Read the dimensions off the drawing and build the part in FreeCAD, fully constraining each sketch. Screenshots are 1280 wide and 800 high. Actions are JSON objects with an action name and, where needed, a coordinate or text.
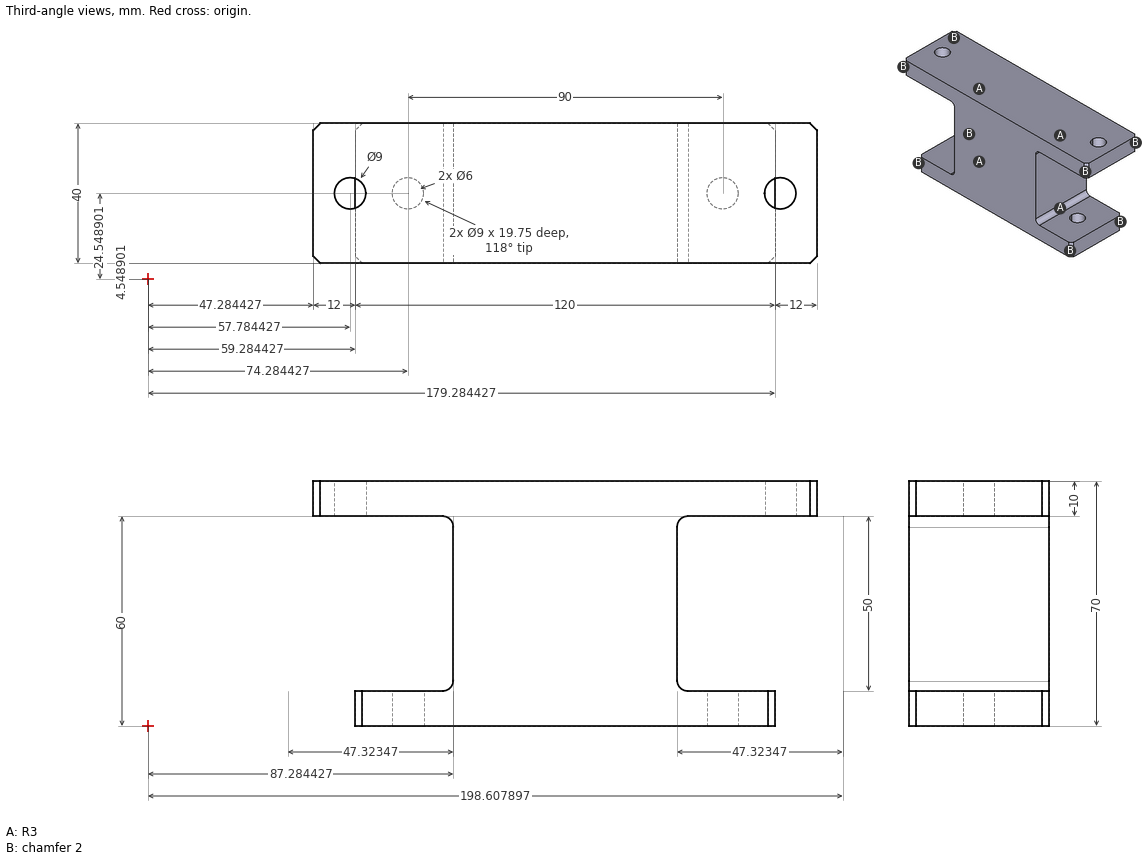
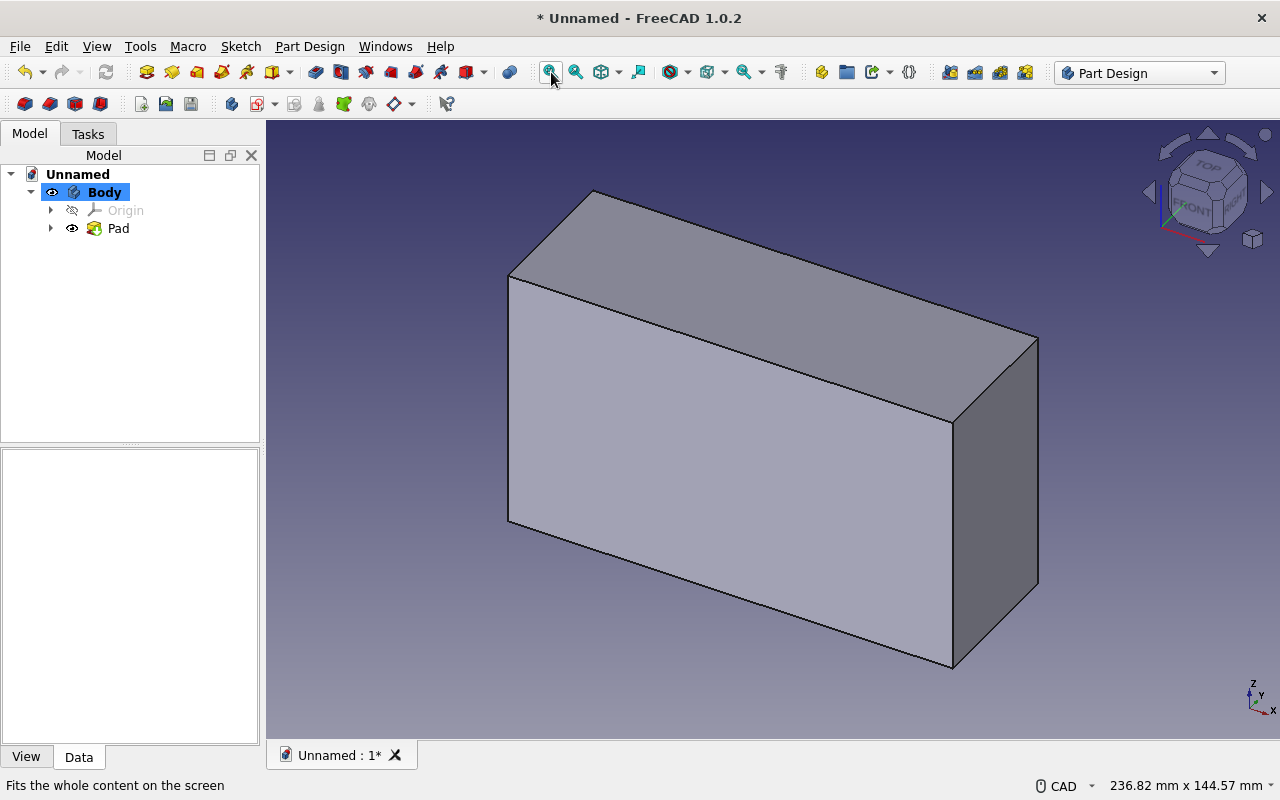
{"action": "left_click", "coordinate": [900, 348]}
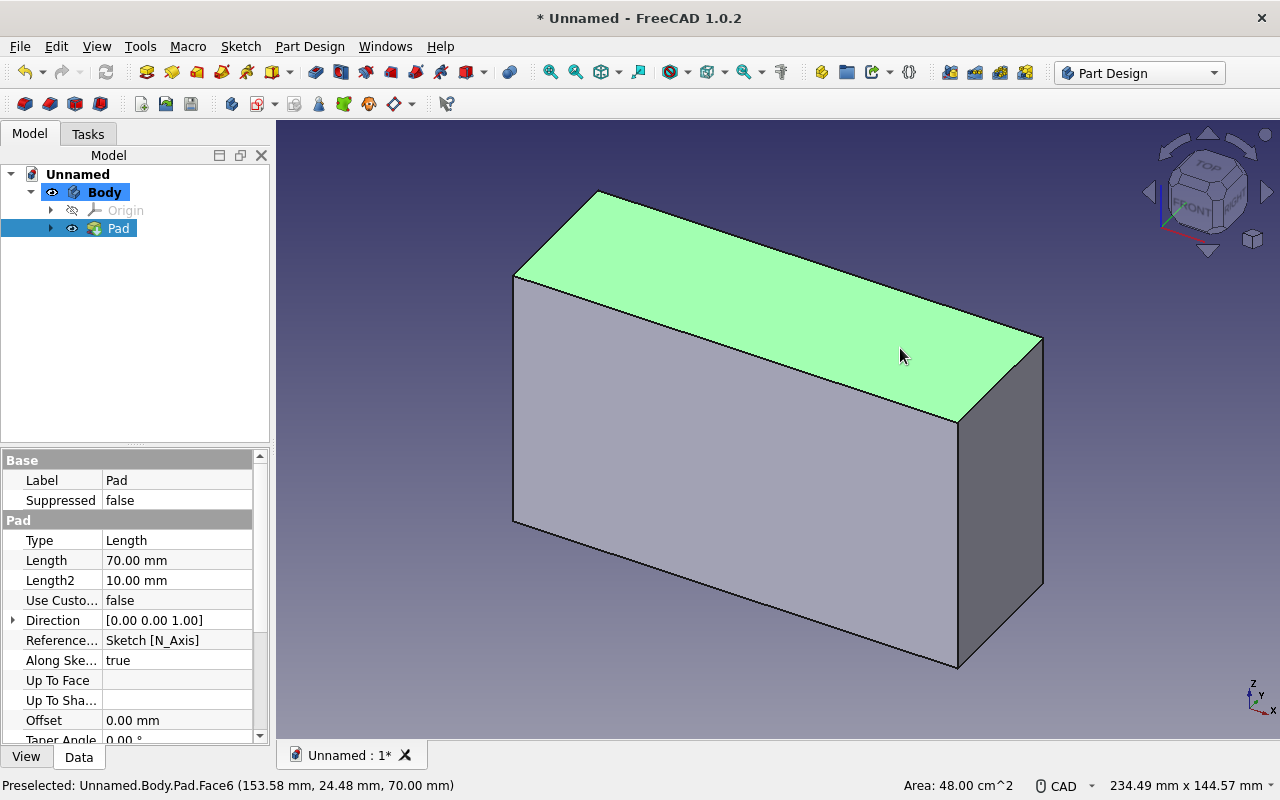
{"action": "left_click", "coordinate": [256, 104]}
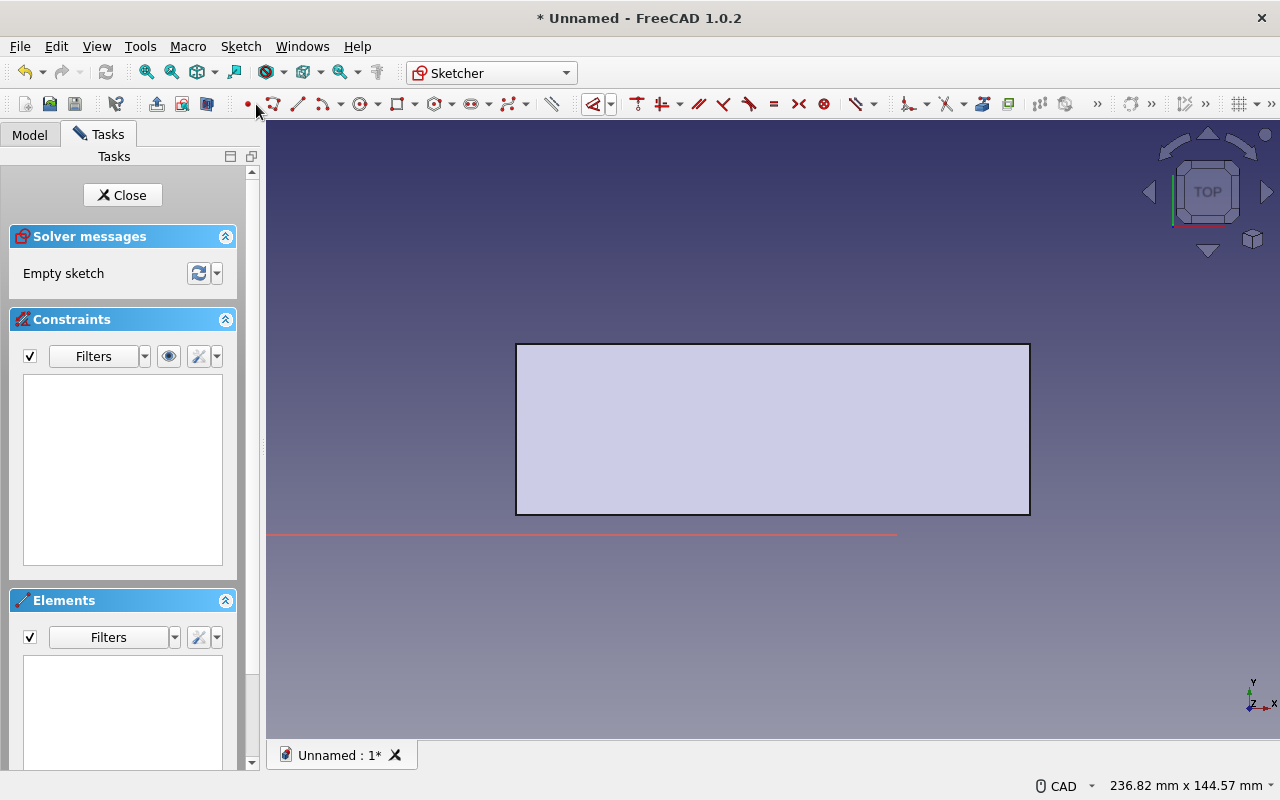
{"action": "scroll", "coordinate": [1084, 221], "scroll_direction": "down", "scroll_amount": 1}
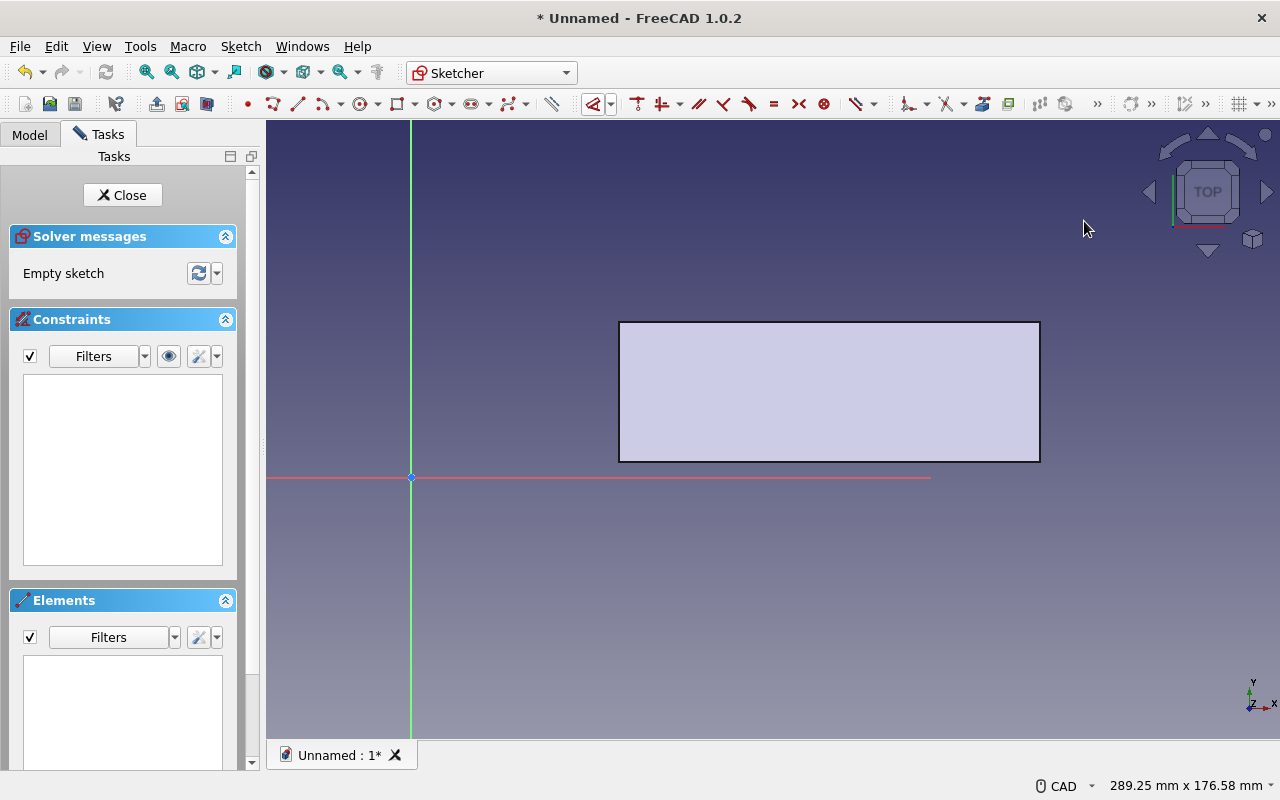
{"action": "key", "text": "g c"}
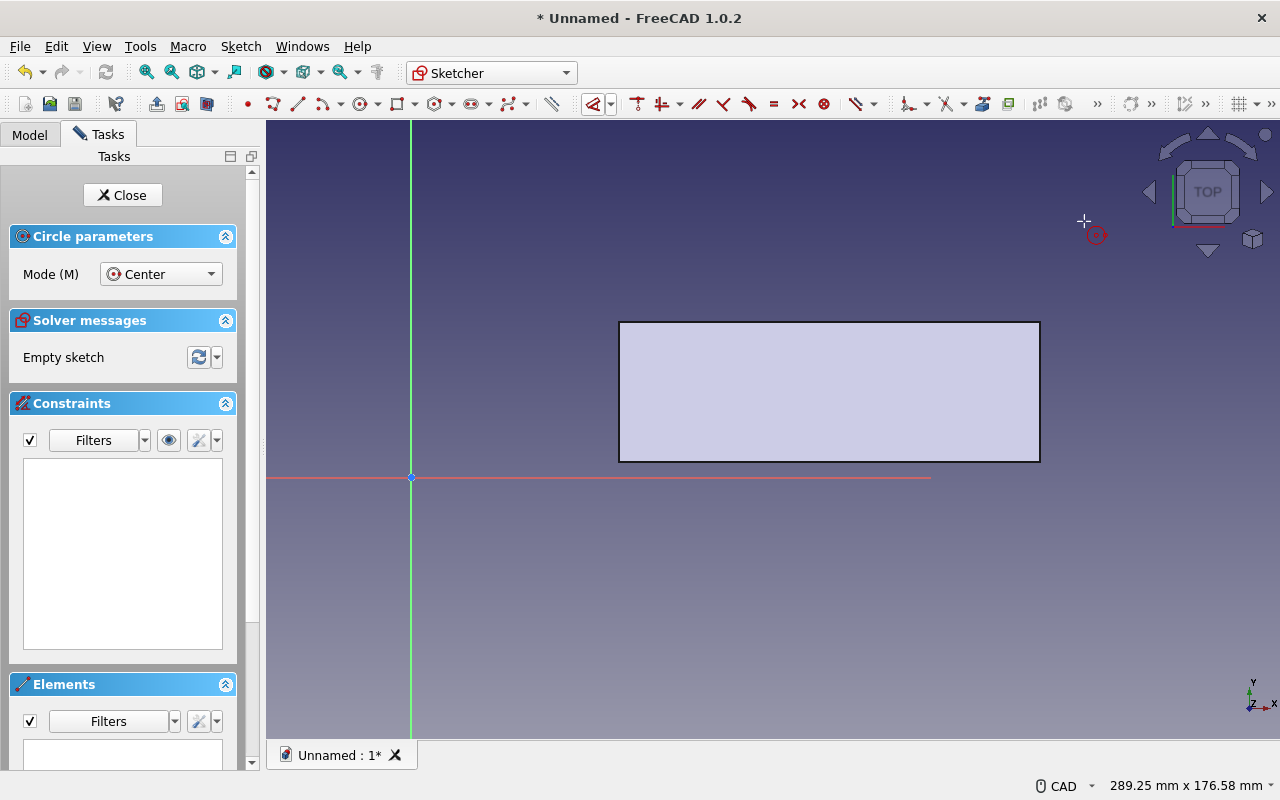
{"action": "scroll", "coordinate": [672, 392], "scroll_direction": "up", "scroll_amount": 4}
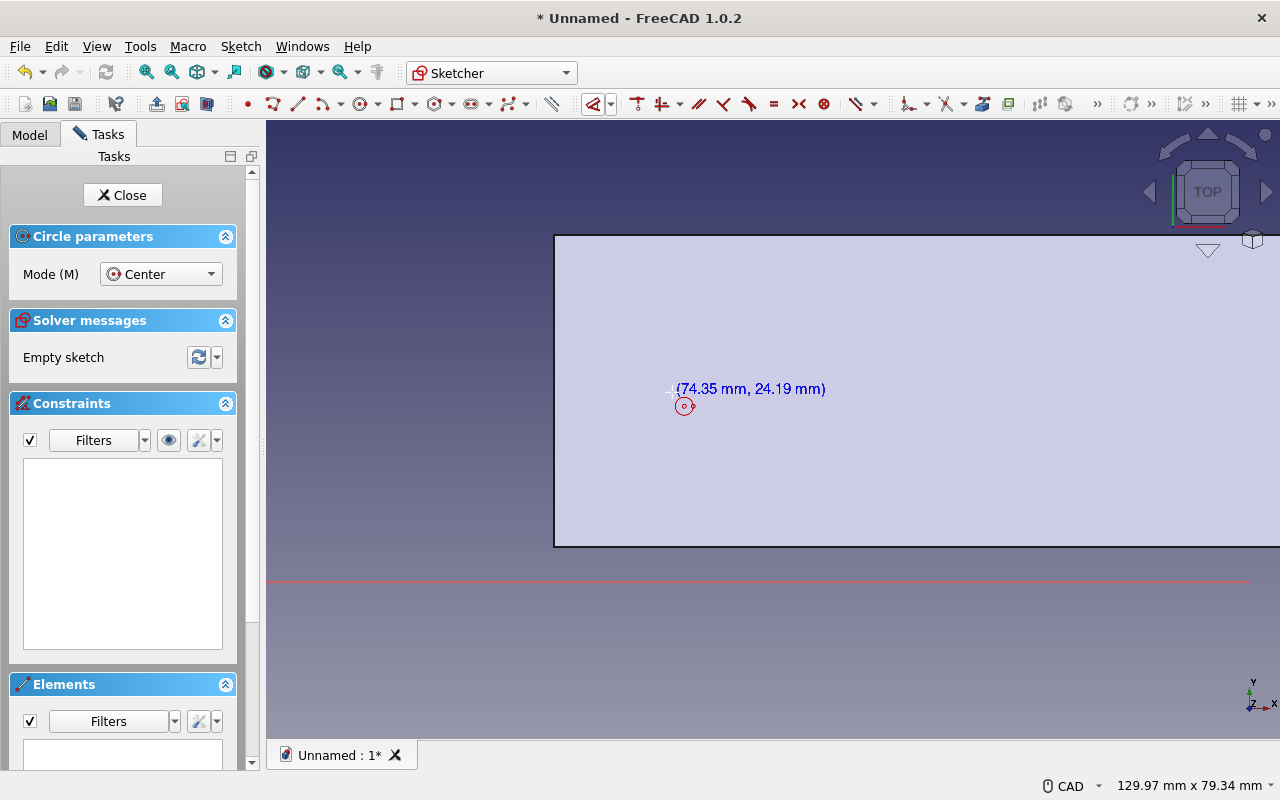
{"action": "left_click", "coordinate": [671, 391]}
{"action": "left_click", "coordinate": [688, 374]}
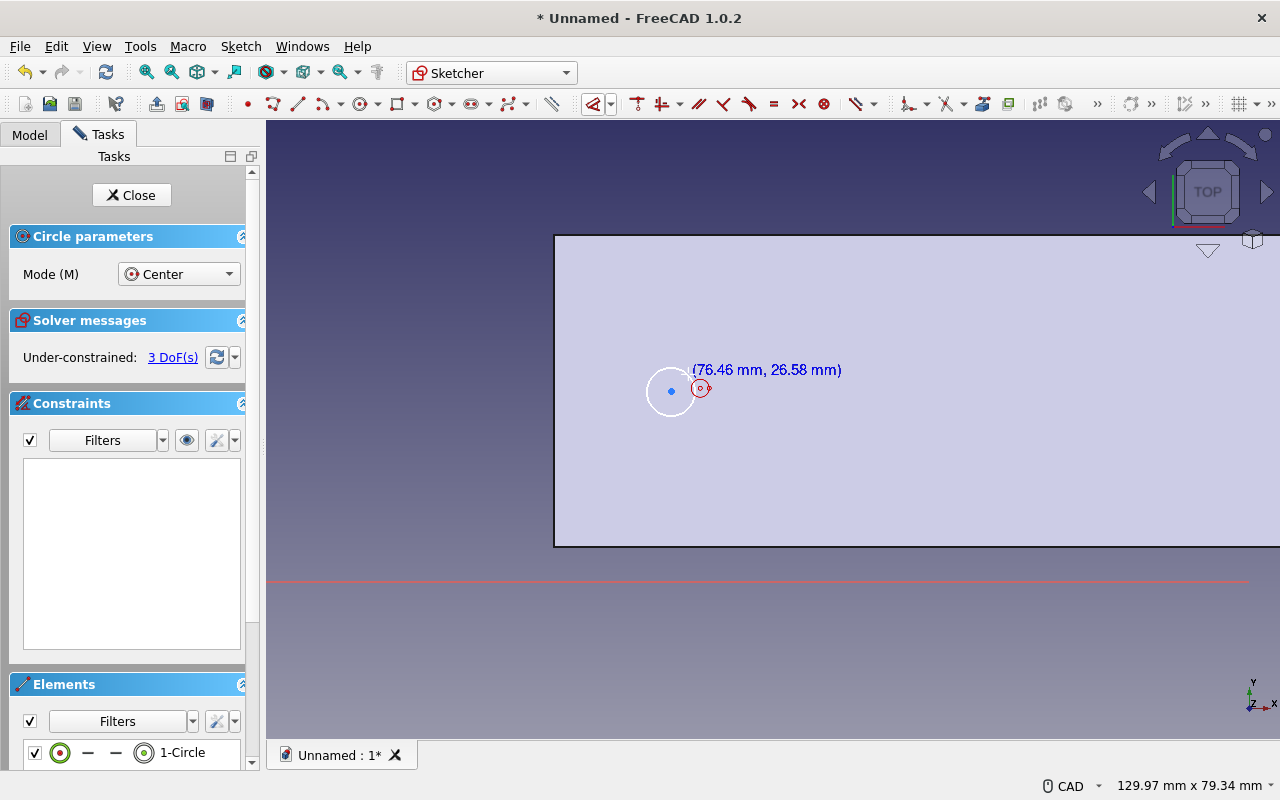
{"action": "scroll", "coordinate": [672, 392], "scroll_direction": "down", "scroll_amount": 4}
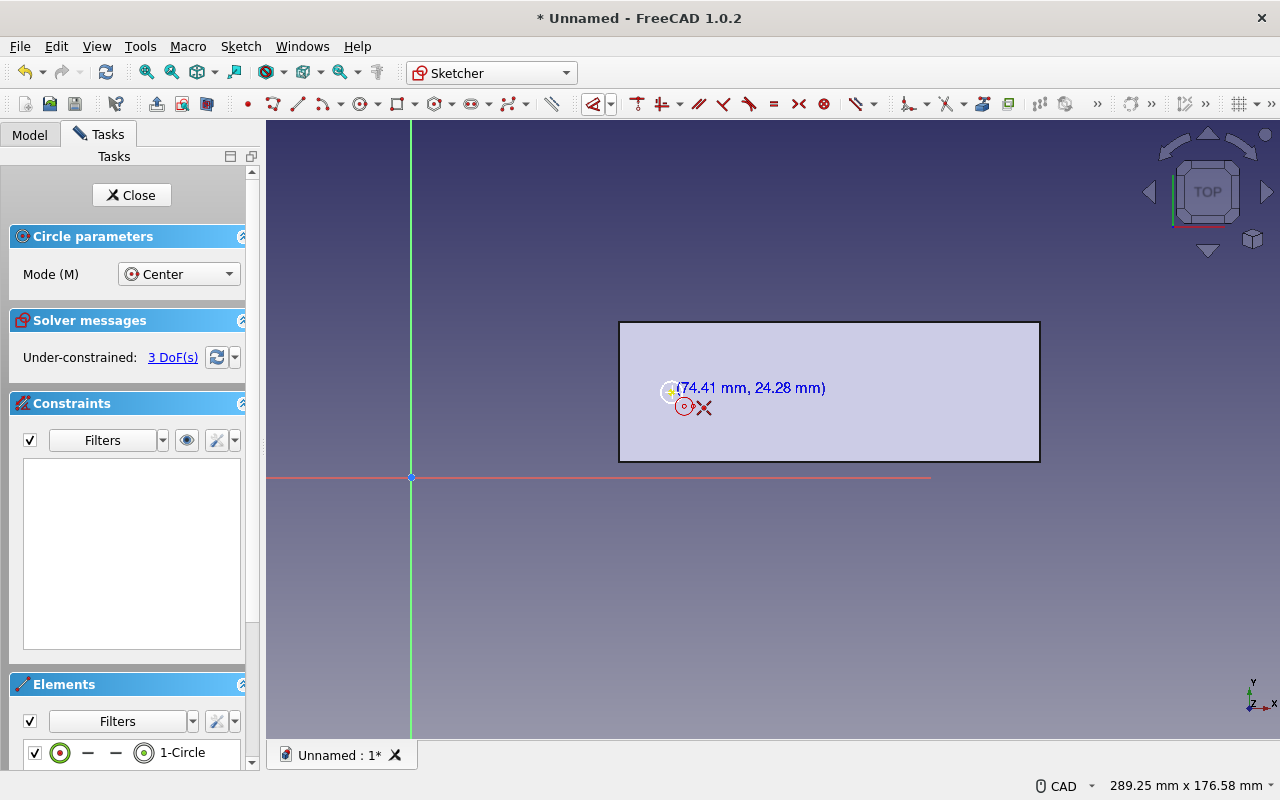
{"action": "scroll", "coordinate": [987, 392], "scroll_direction": "up", "scroll_amount": 4}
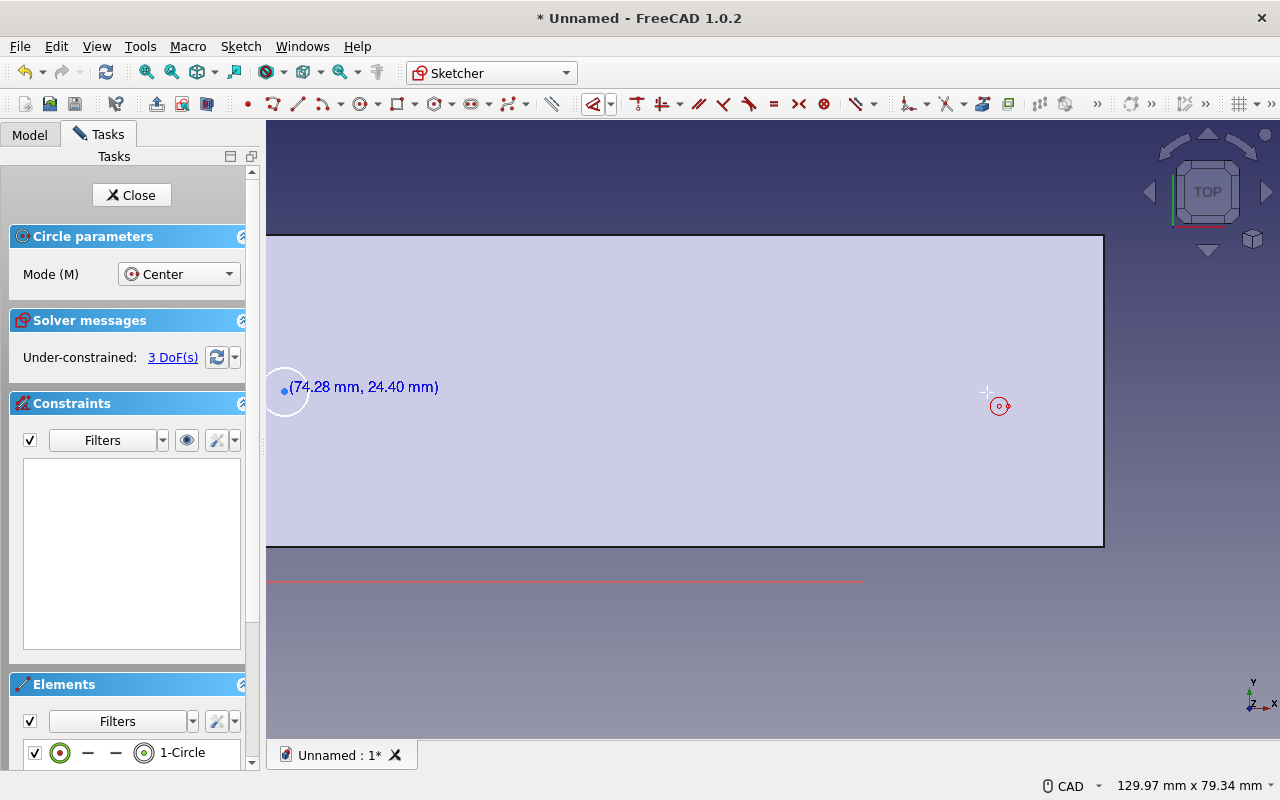
{"action": "left_click", "coordinate": [987, 391]}
{"action": "left_click", "coordinate": [1003, 374]}
{"action": "key", "text": "Escape"}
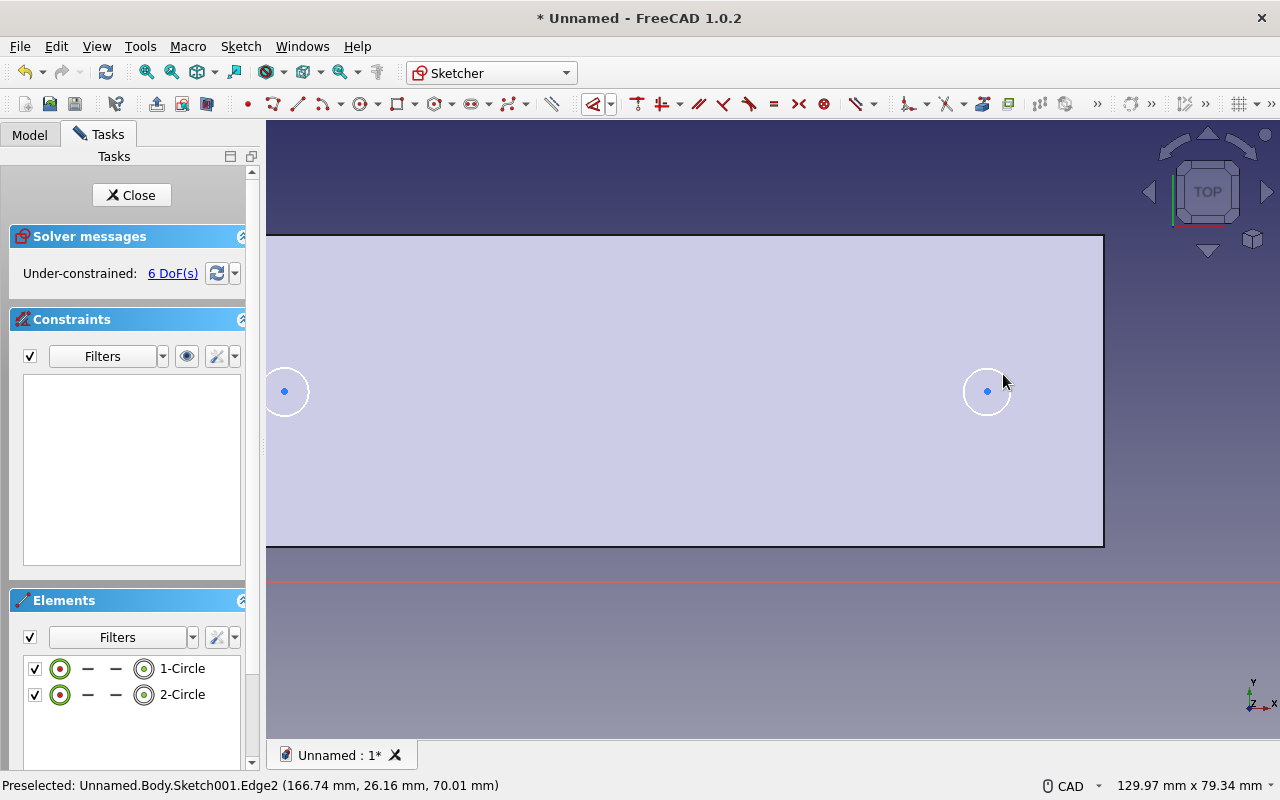
{"action": "left_click", "coordinate": [302, 375]}